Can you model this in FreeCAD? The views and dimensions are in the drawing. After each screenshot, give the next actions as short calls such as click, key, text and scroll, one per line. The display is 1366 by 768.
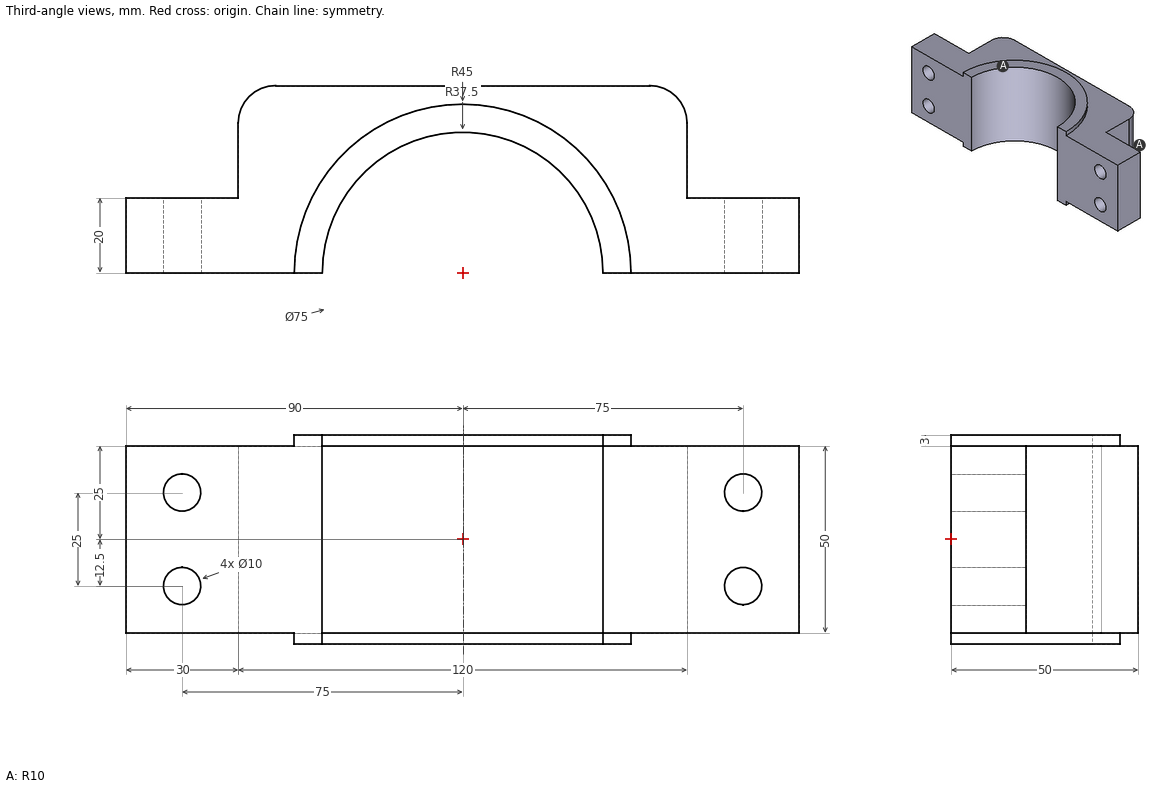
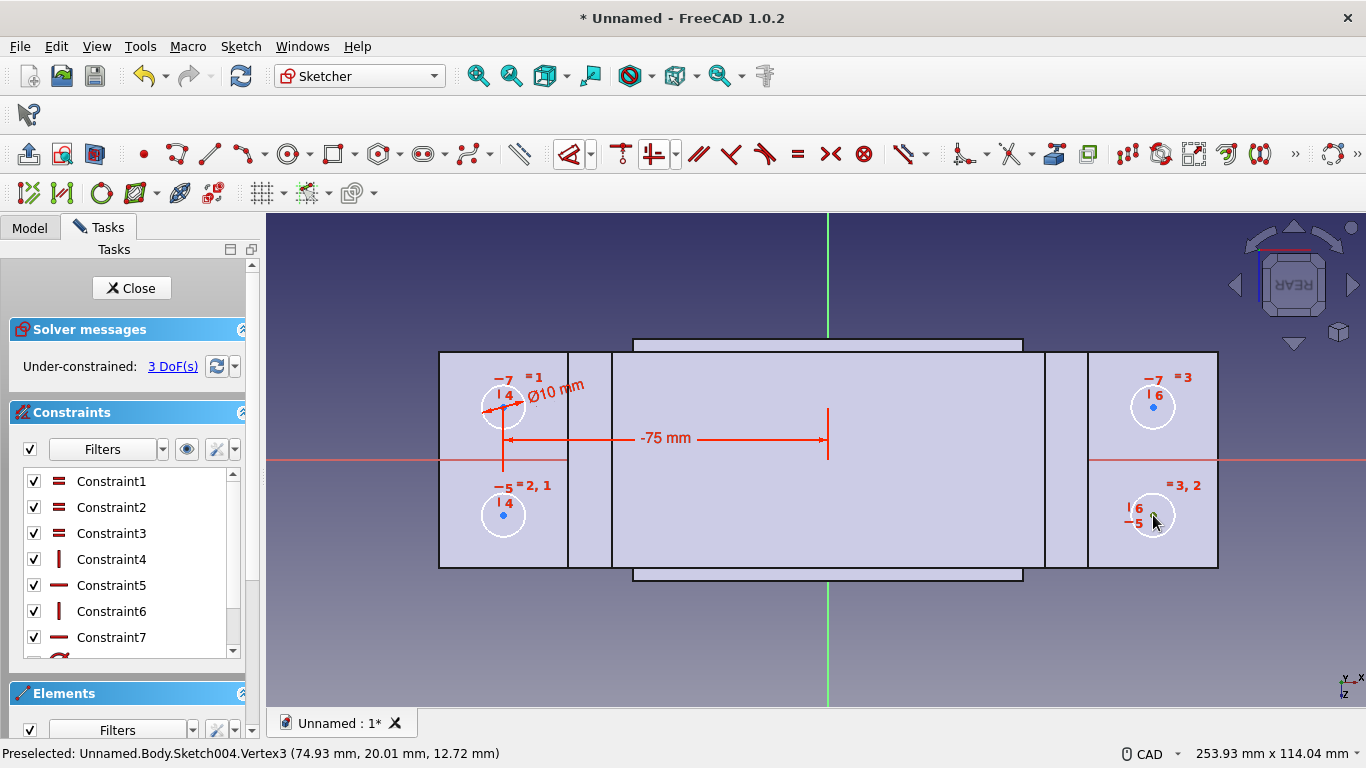
key(l)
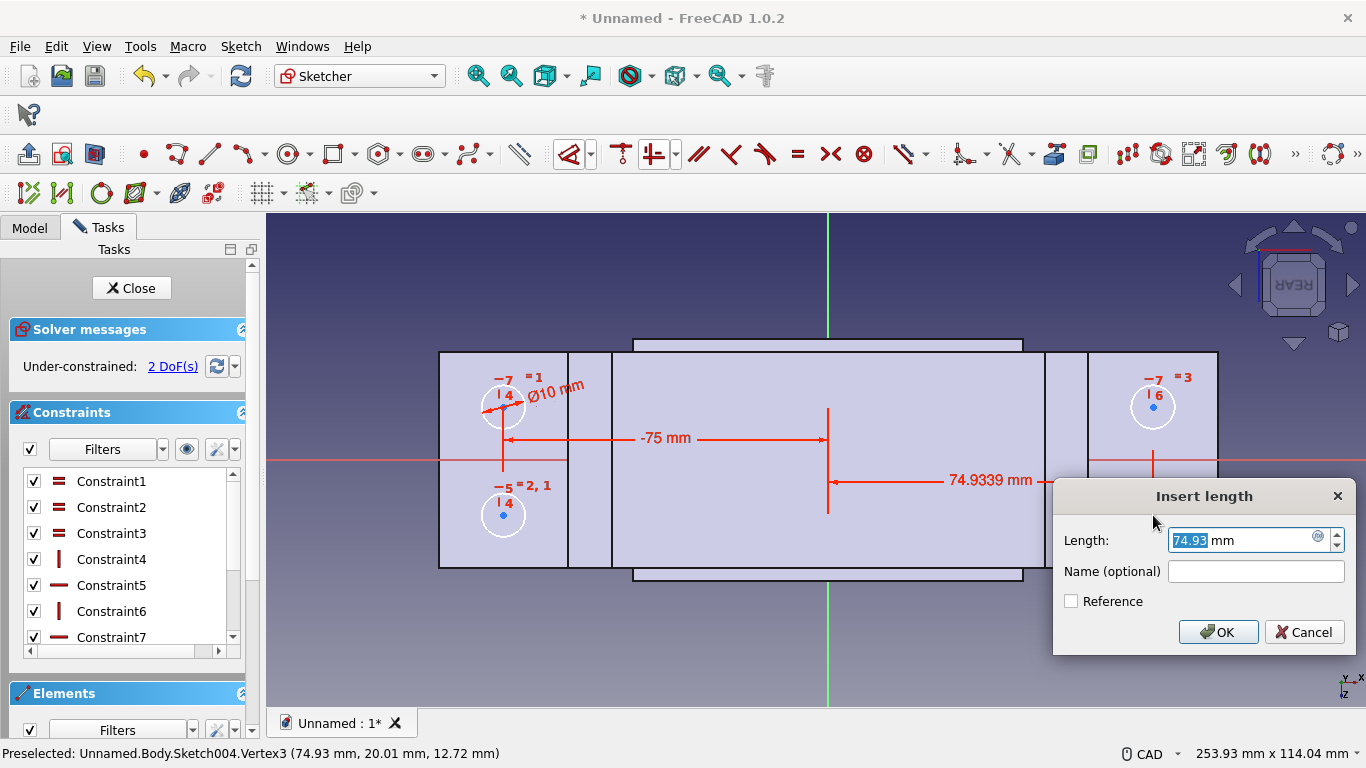
text(75)
key(Return)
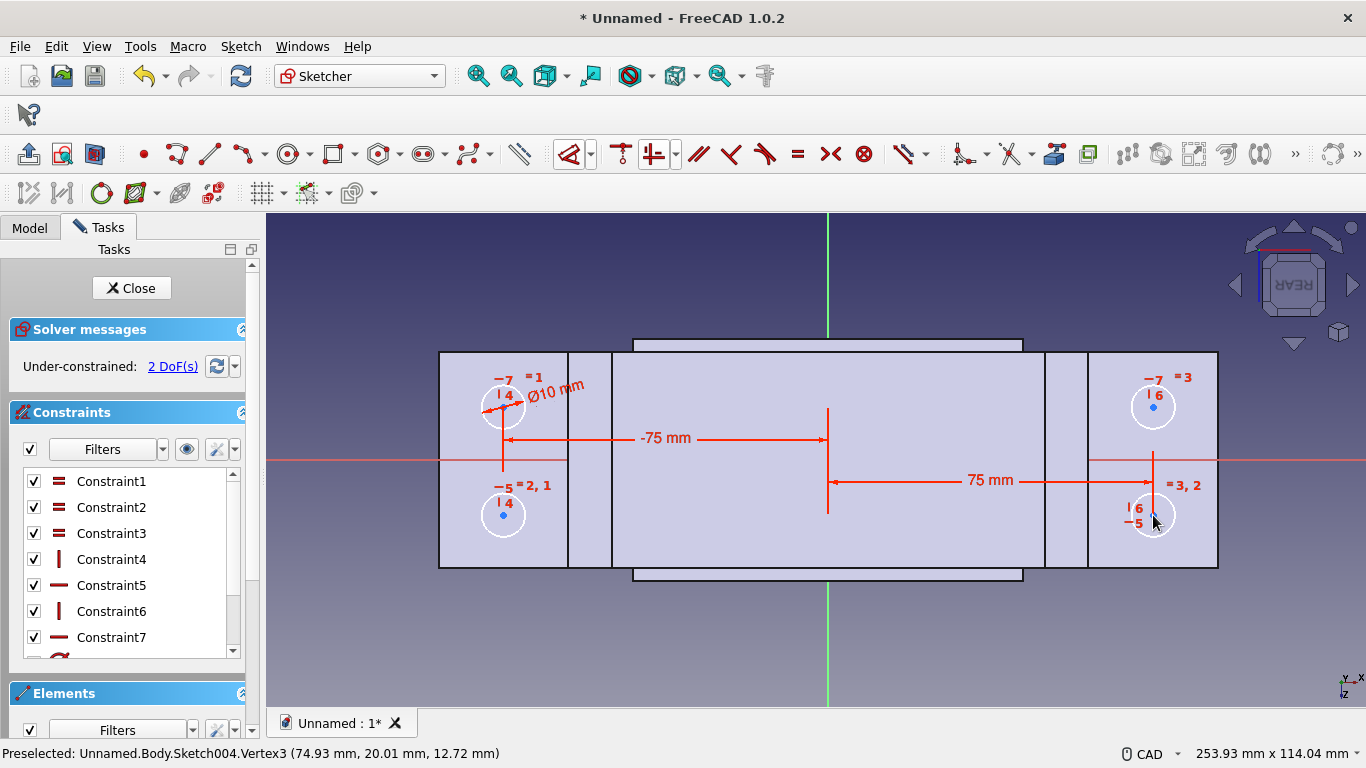
click(503, 407)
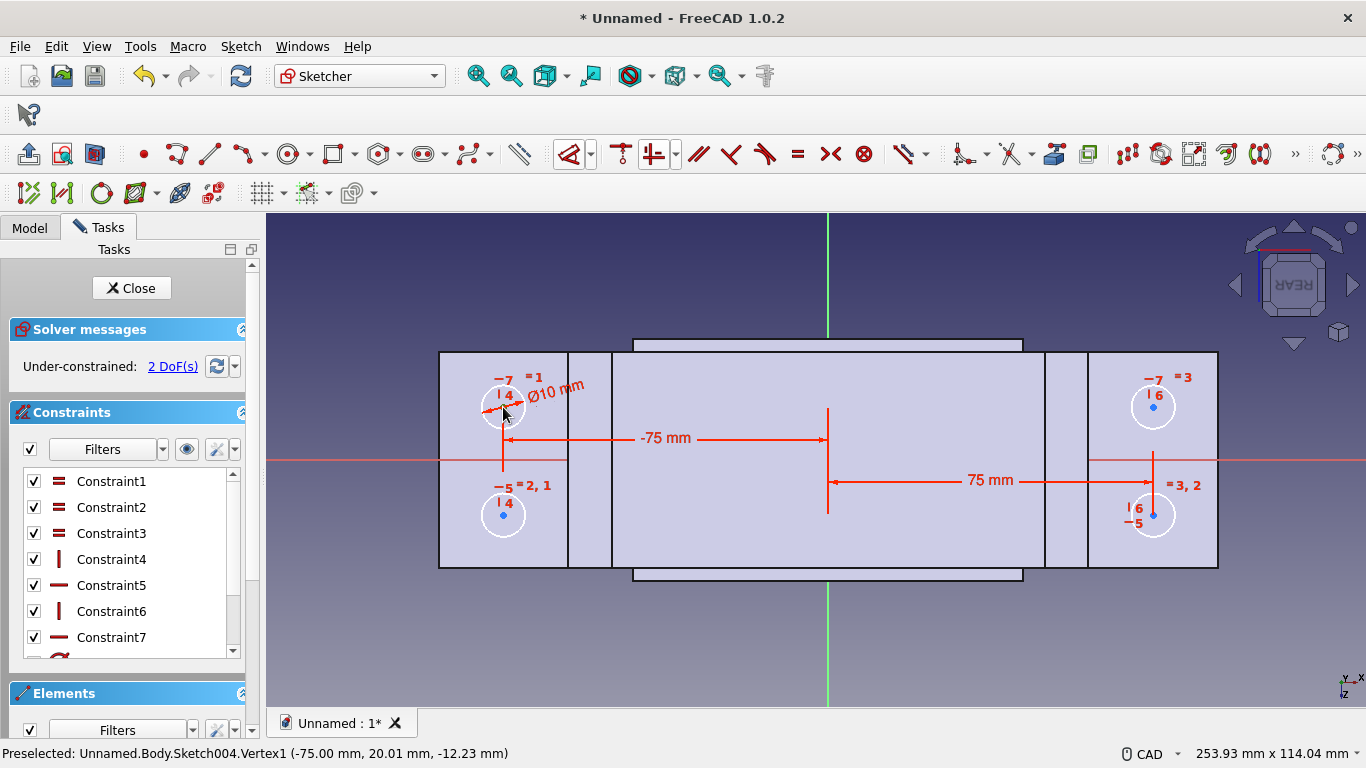
click(503, 515)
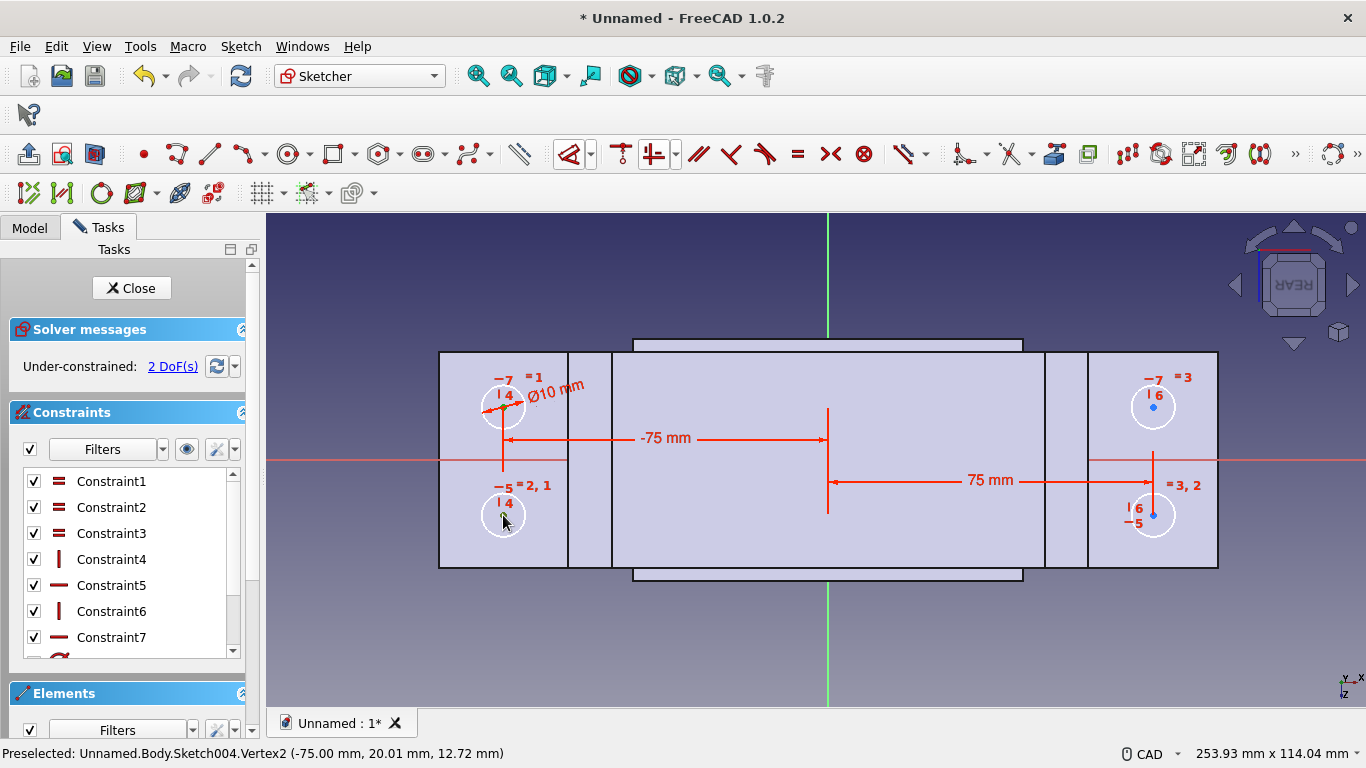
key(i)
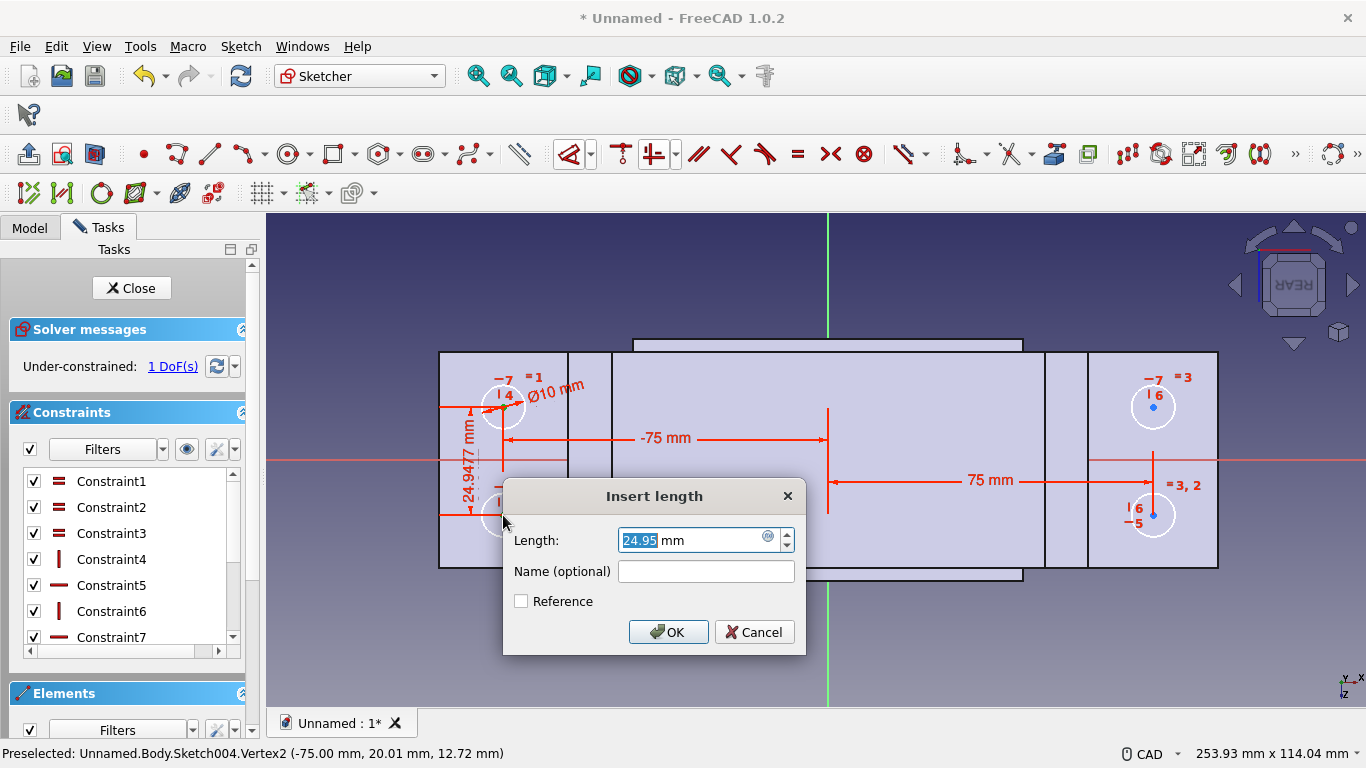
text(25)
key(Return)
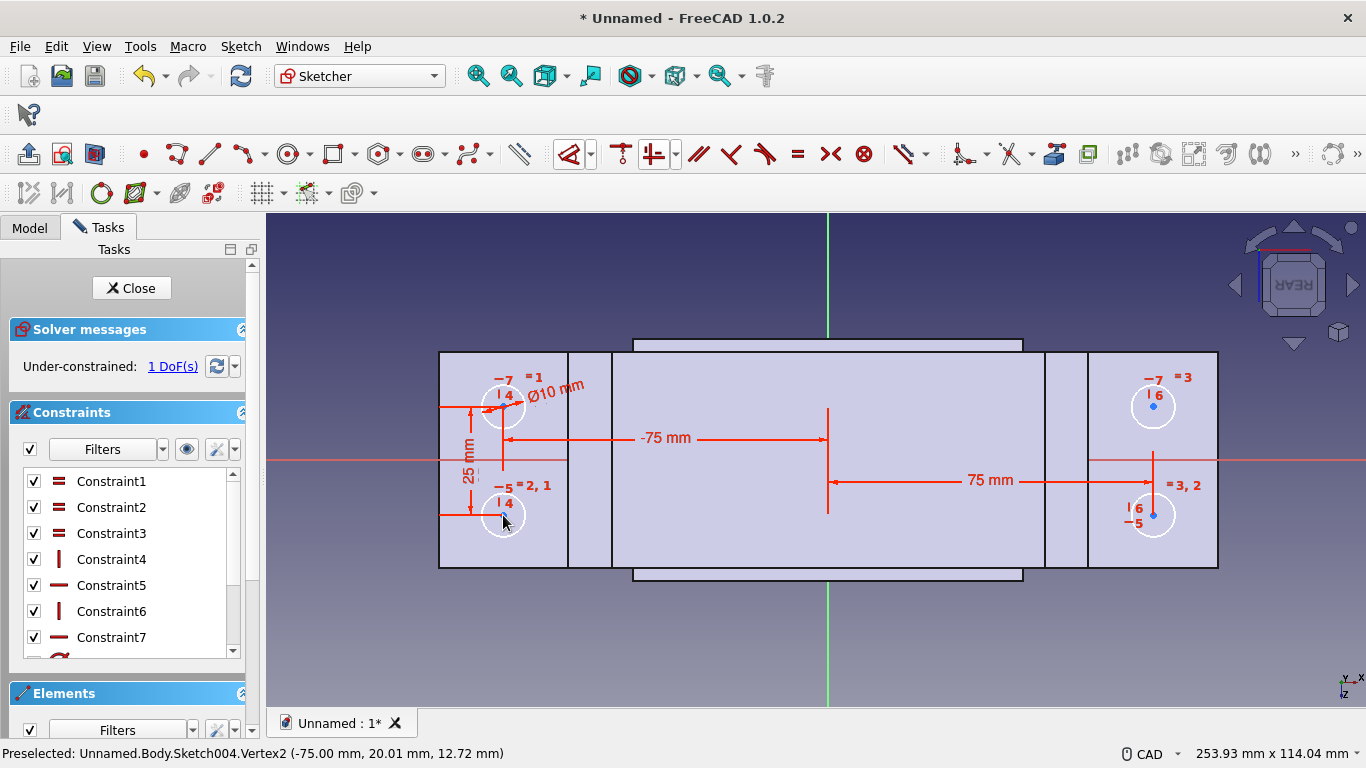
click(503, 407)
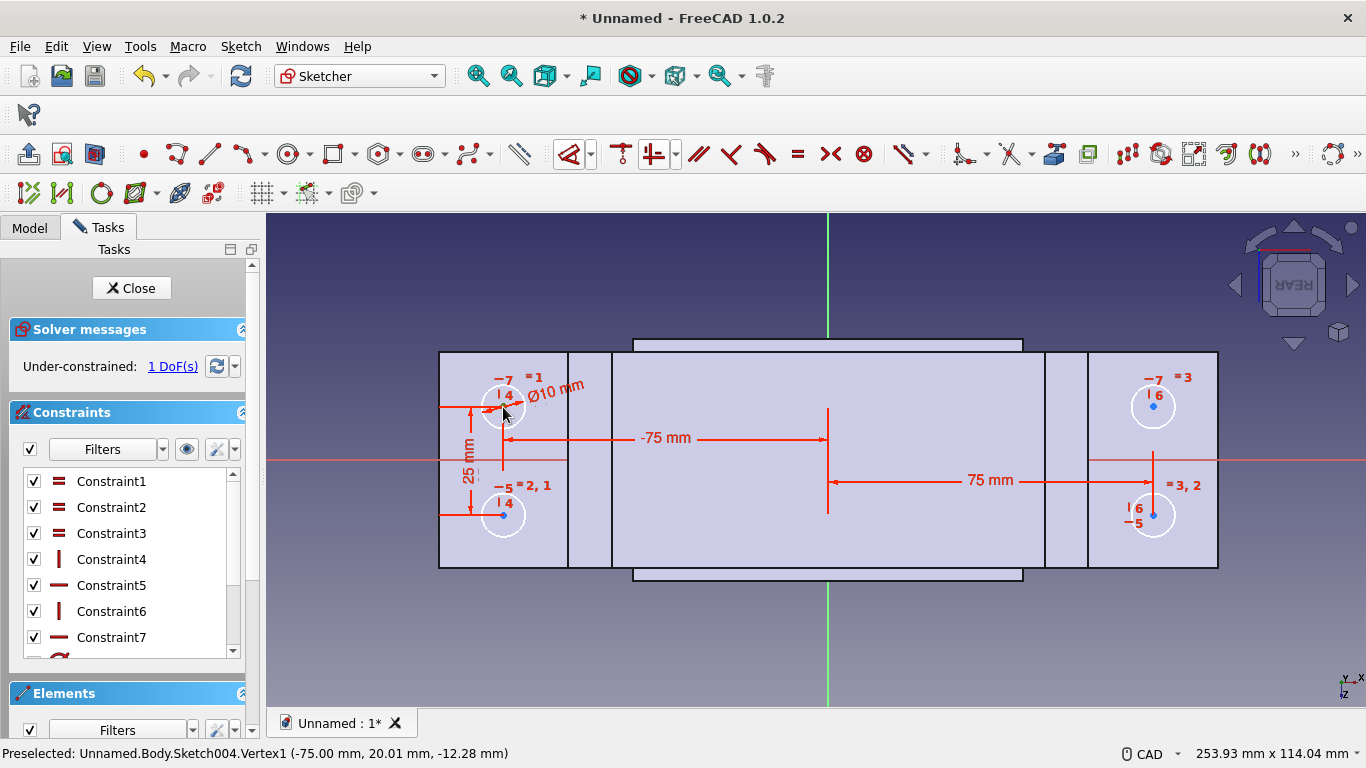
click(590, 154)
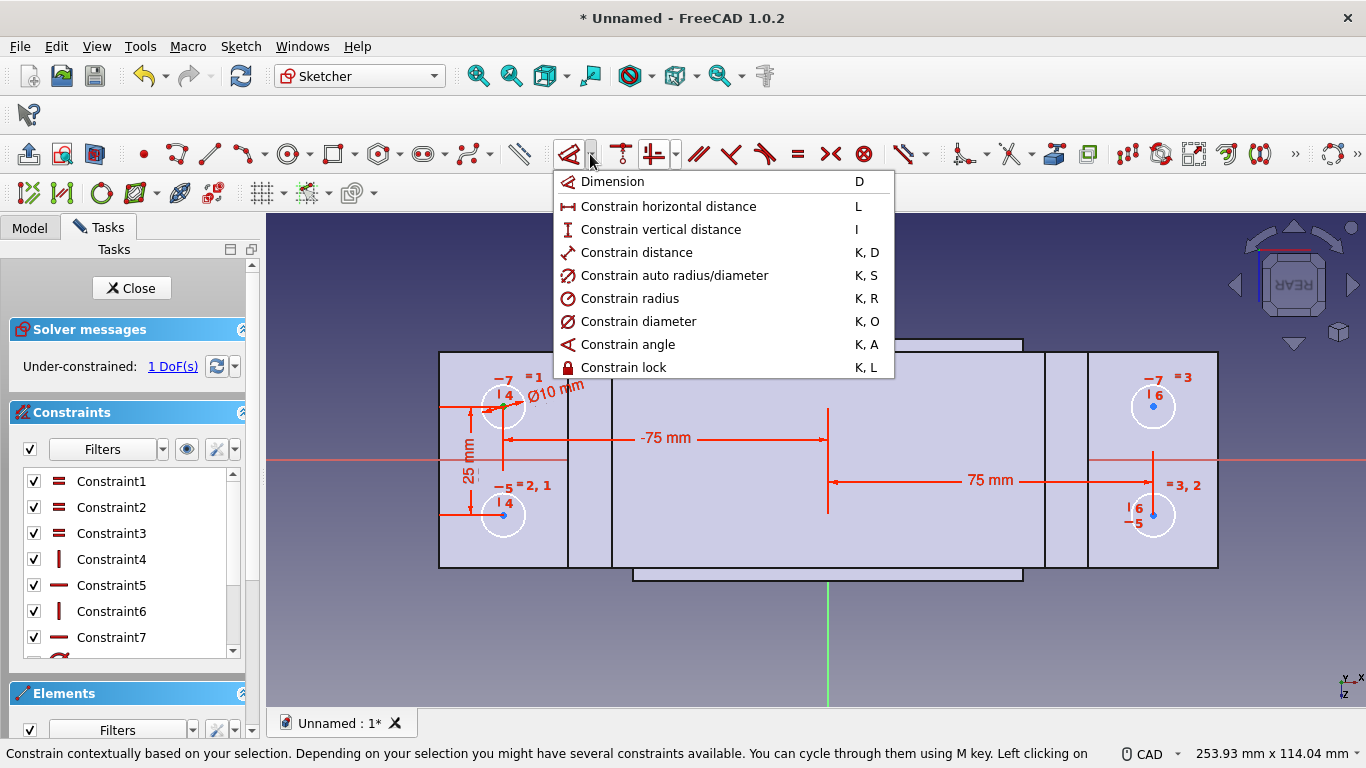
click(724, 230)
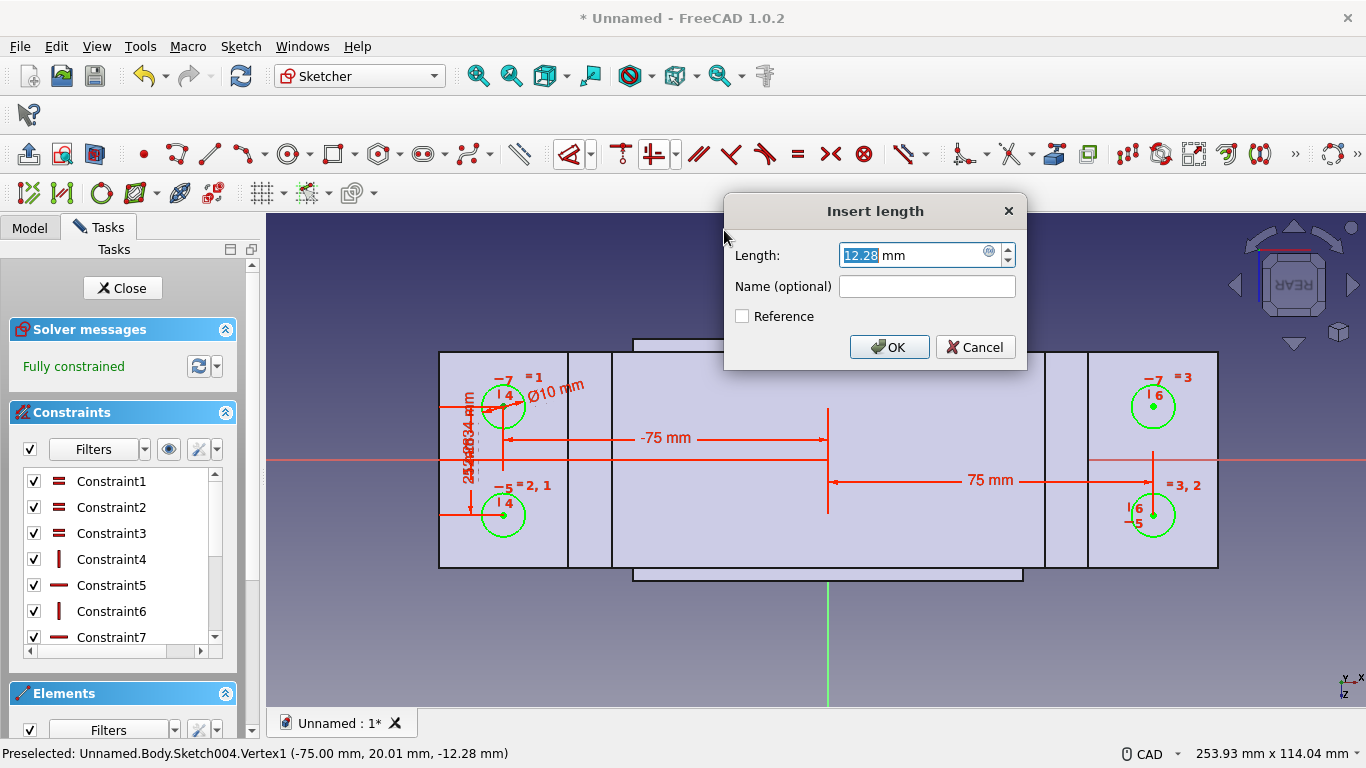
text(12.5)
key(Return)